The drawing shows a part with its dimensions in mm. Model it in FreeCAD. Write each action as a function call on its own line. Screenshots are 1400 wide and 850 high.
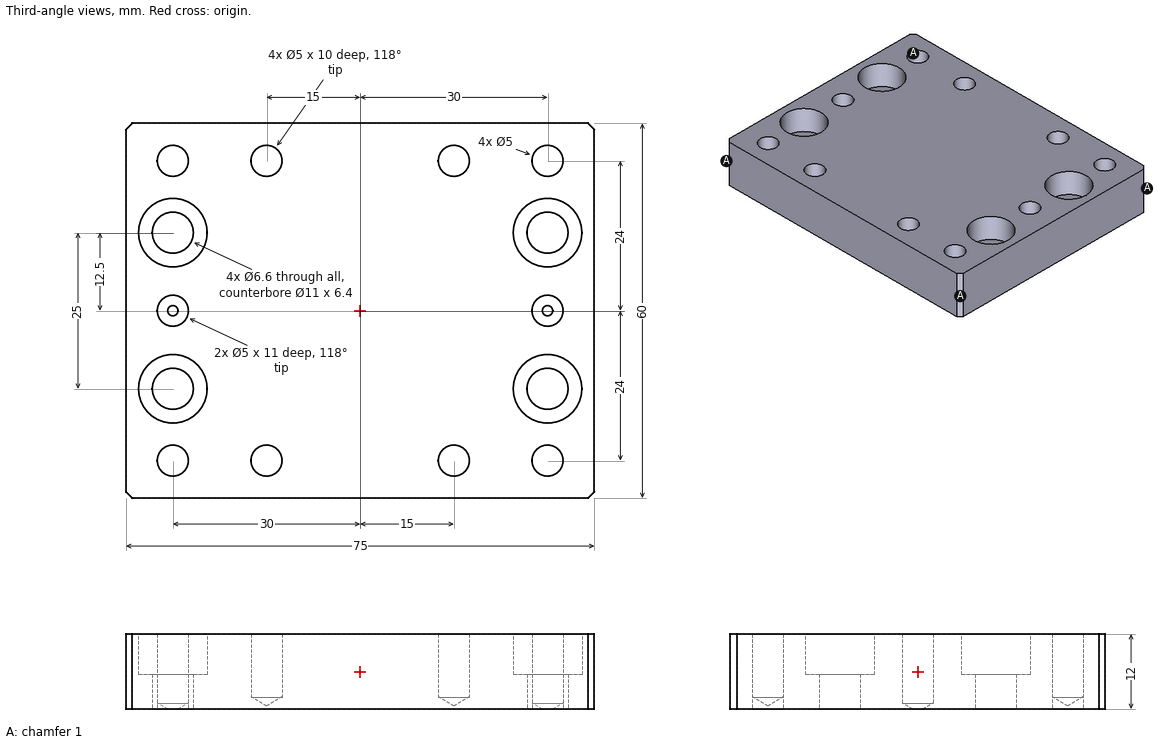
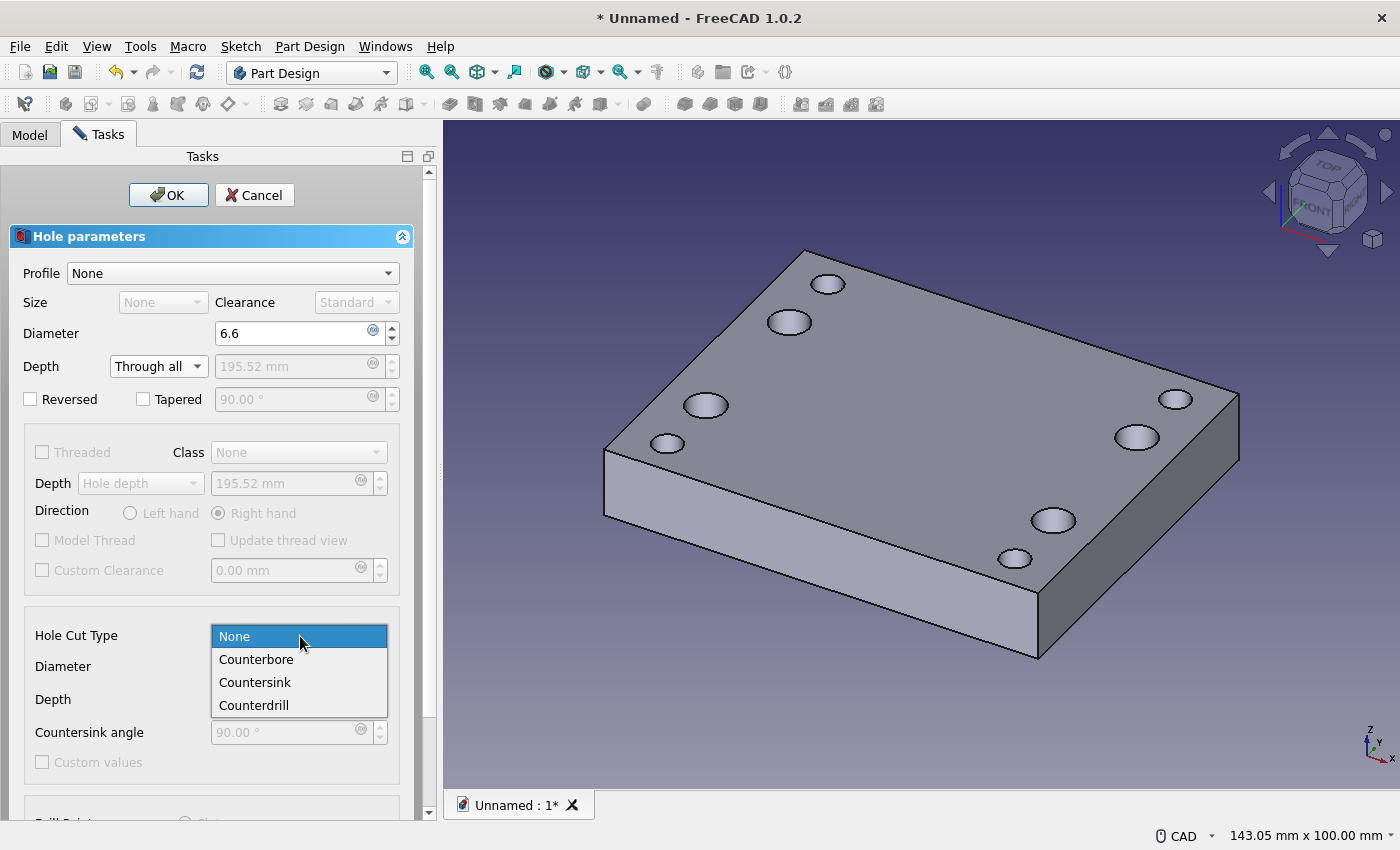
click(298, 660)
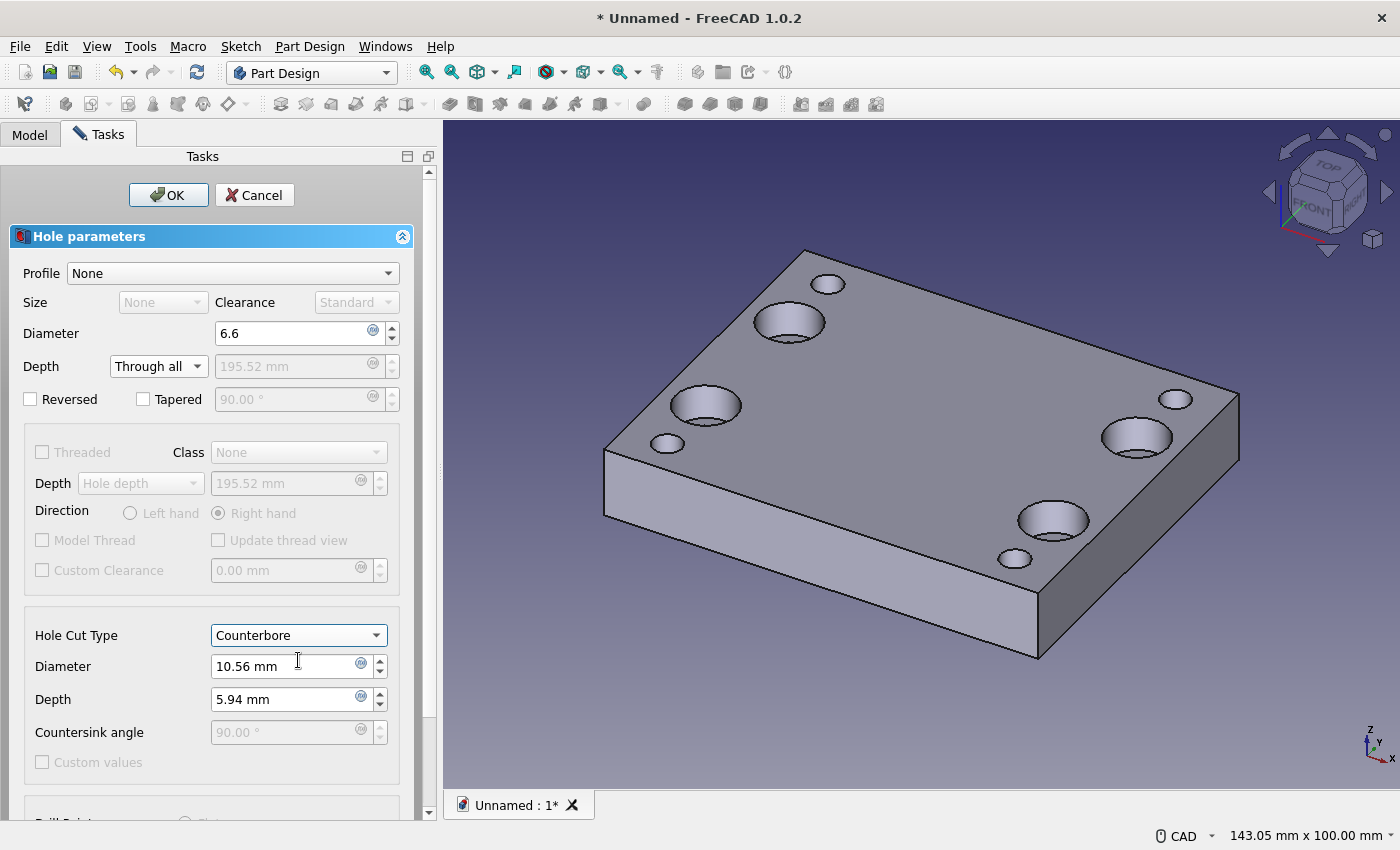
triple_click(292, 666)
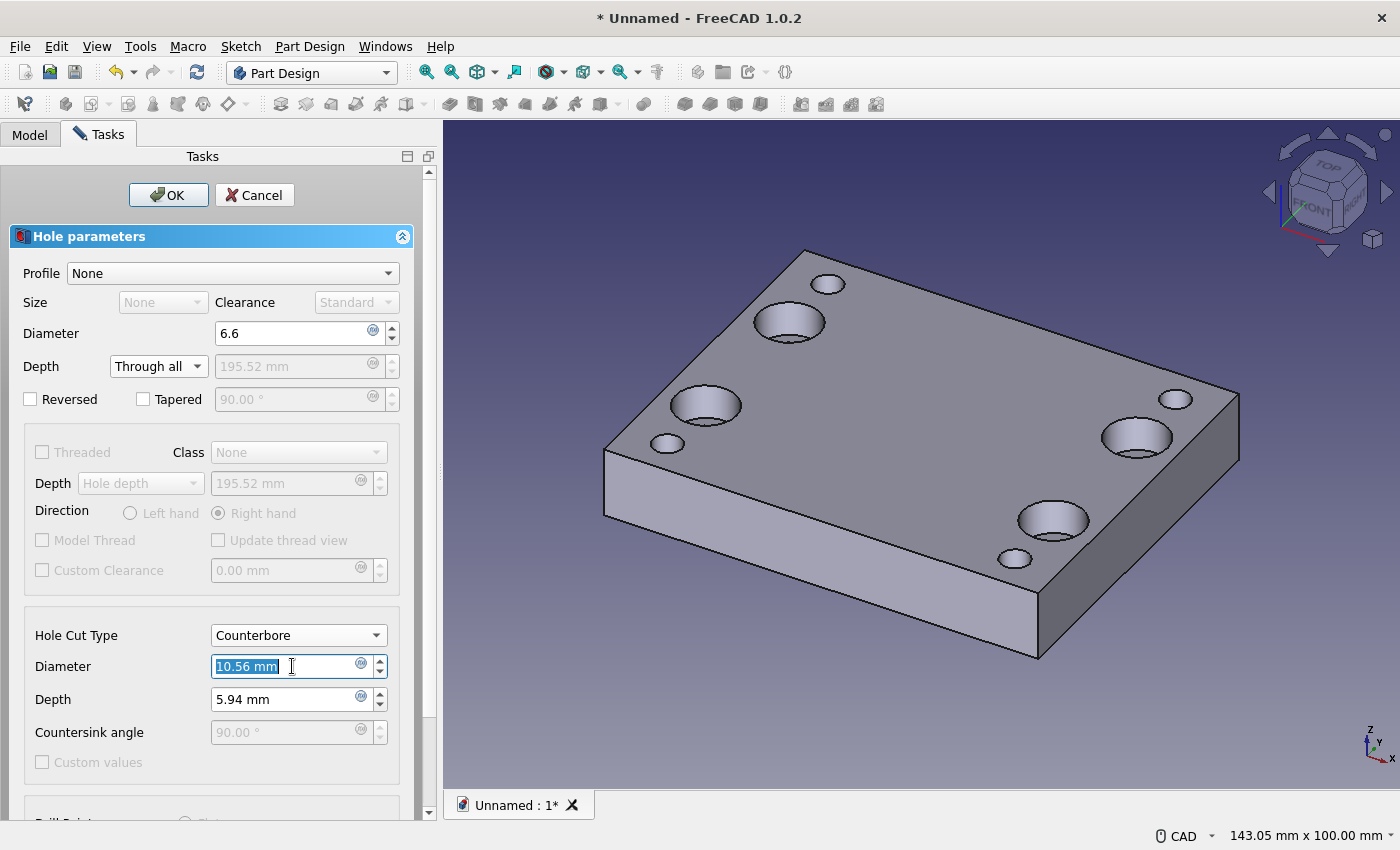
text(11)
key(Tab)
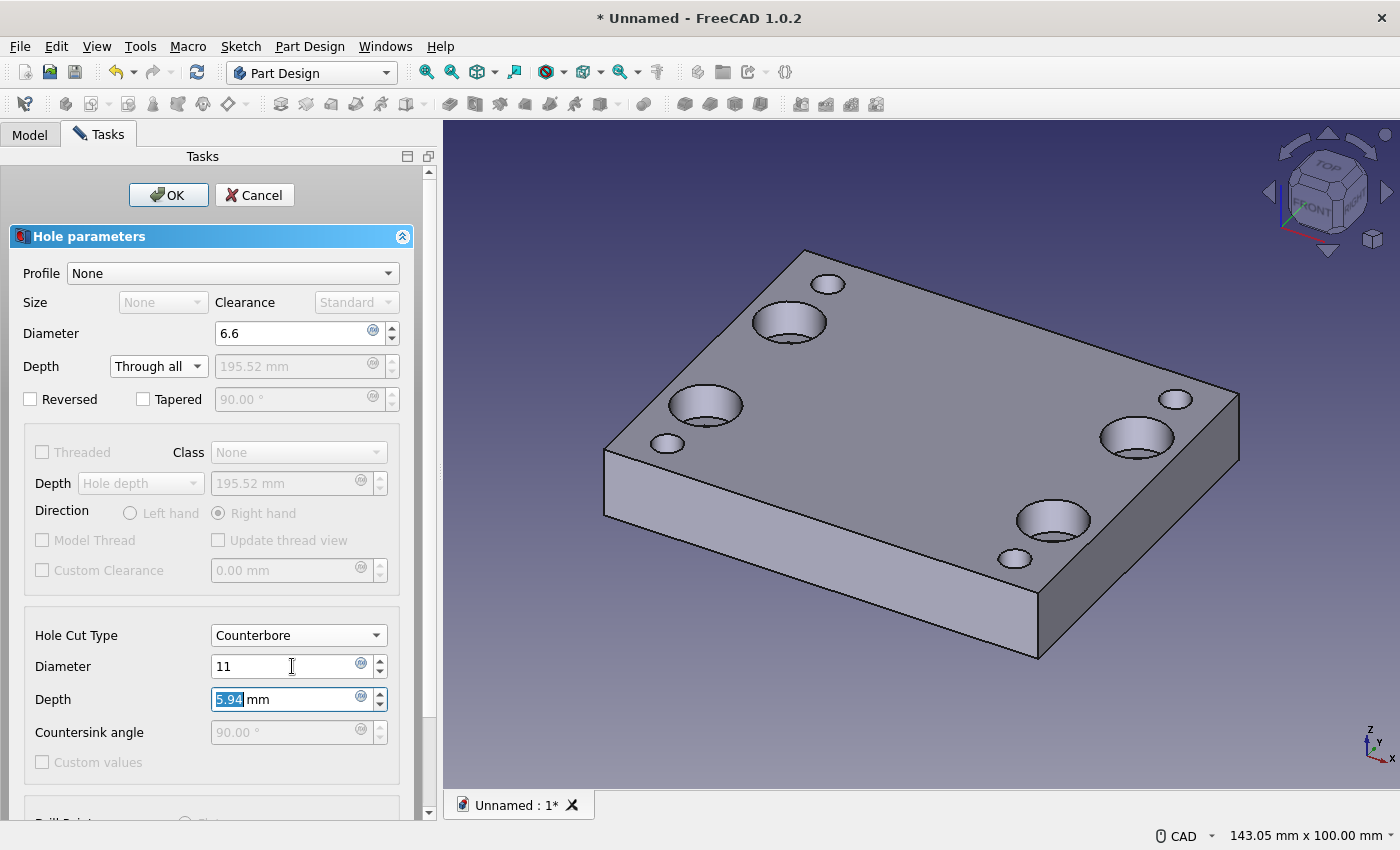
text(6.4)
key(Tab)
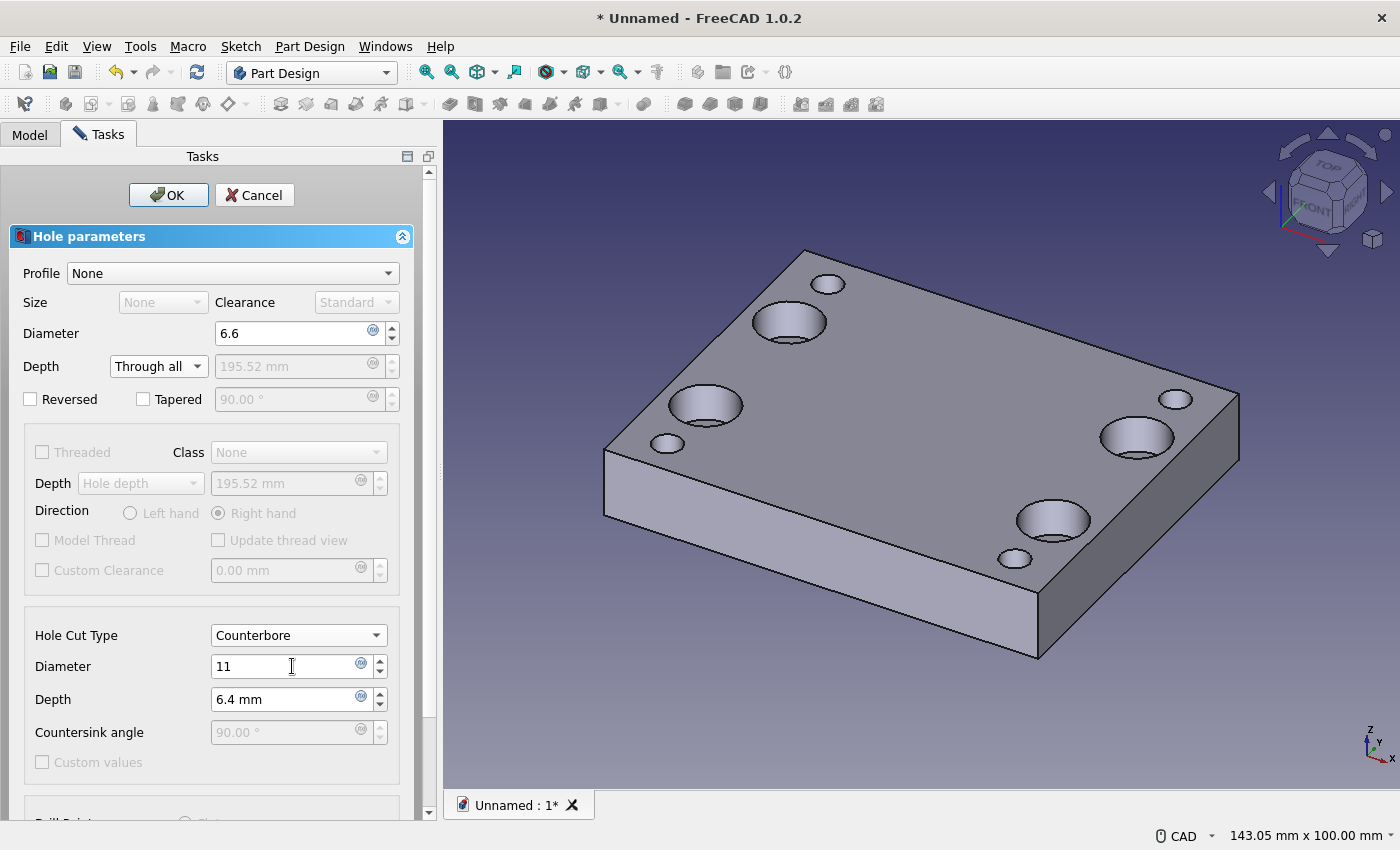
click(169, 195)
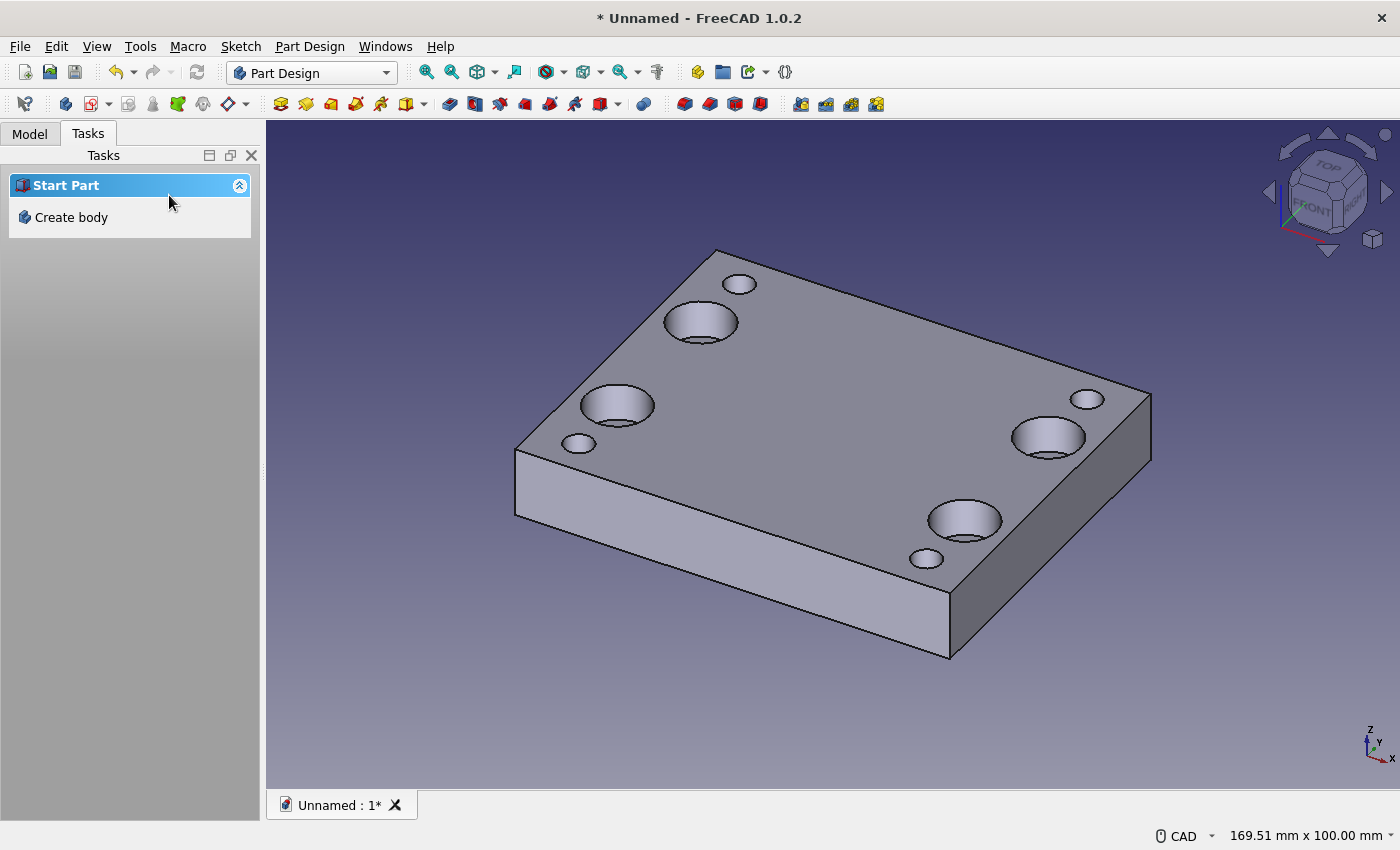
click(833, 421)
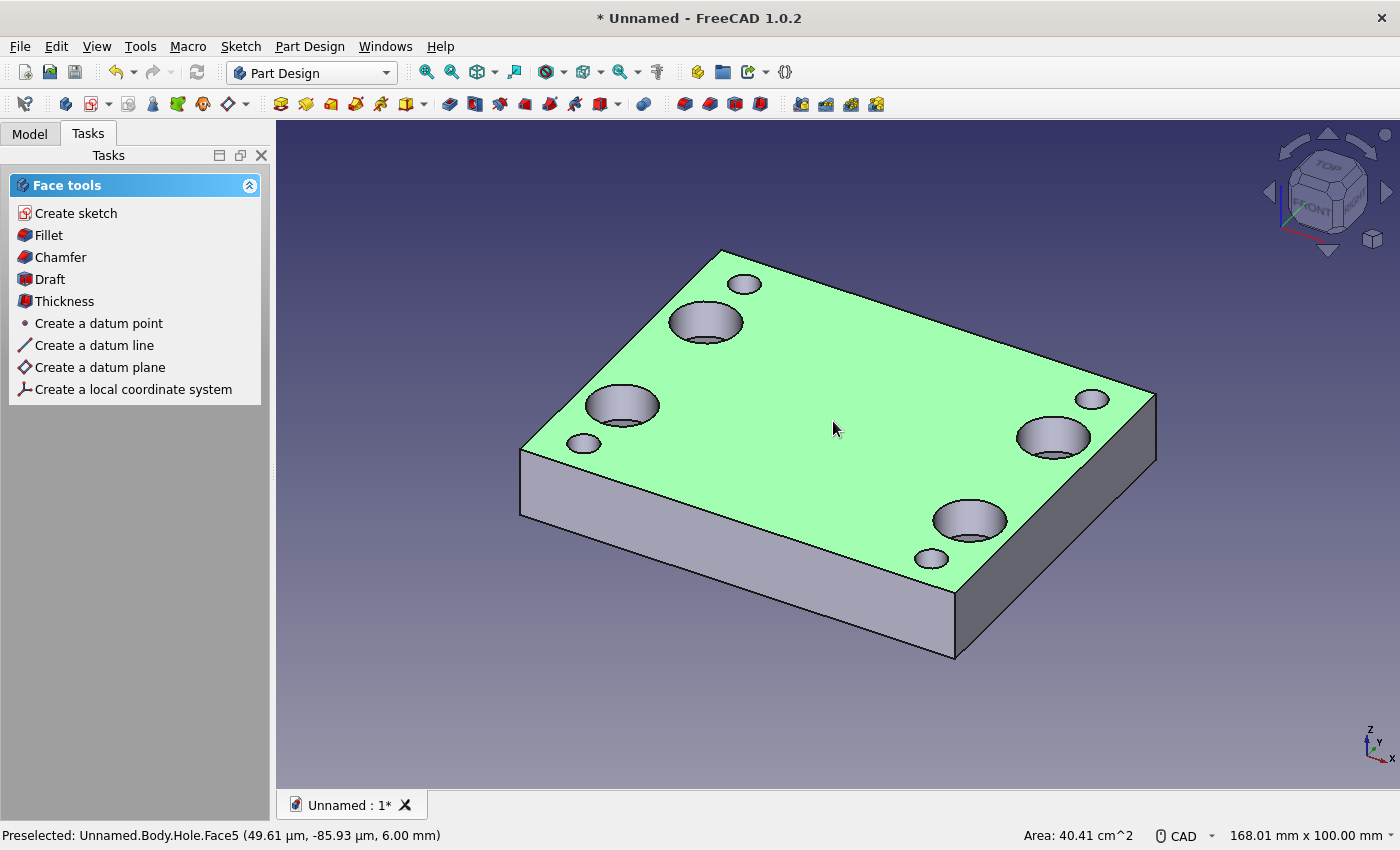
click(90, 104)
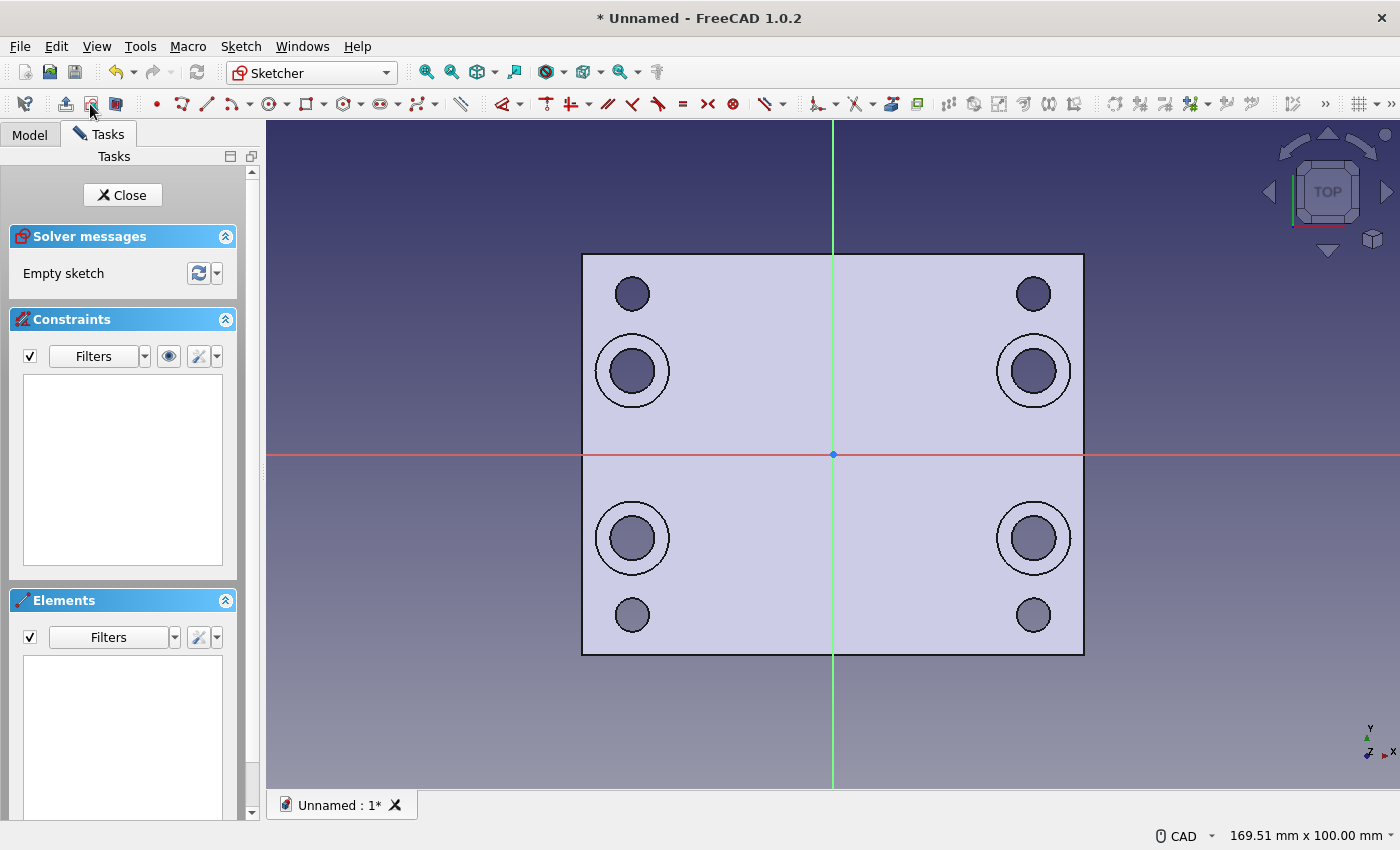
scroll(972, 455, up, 2)